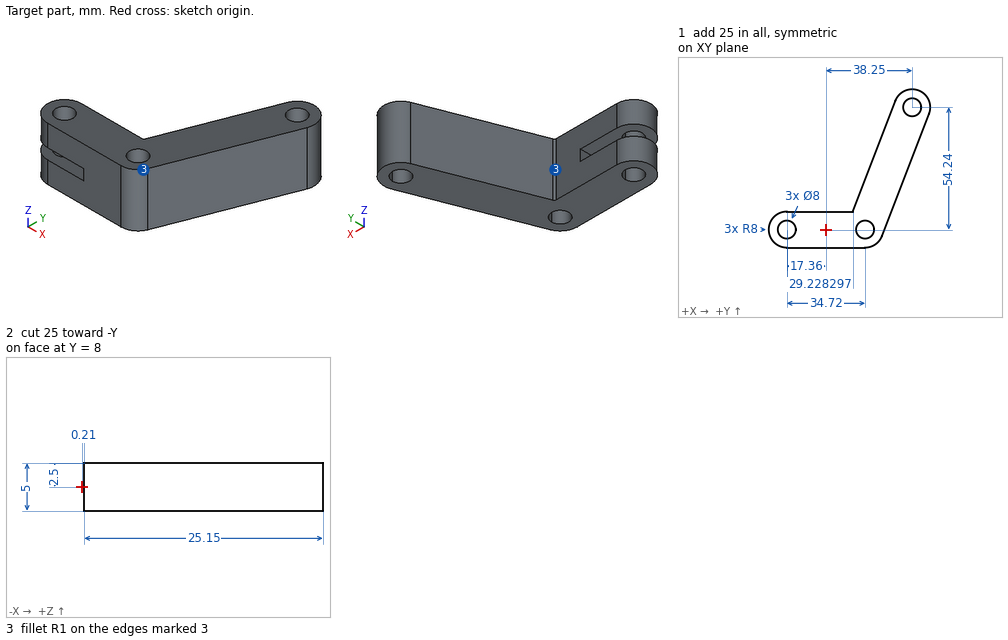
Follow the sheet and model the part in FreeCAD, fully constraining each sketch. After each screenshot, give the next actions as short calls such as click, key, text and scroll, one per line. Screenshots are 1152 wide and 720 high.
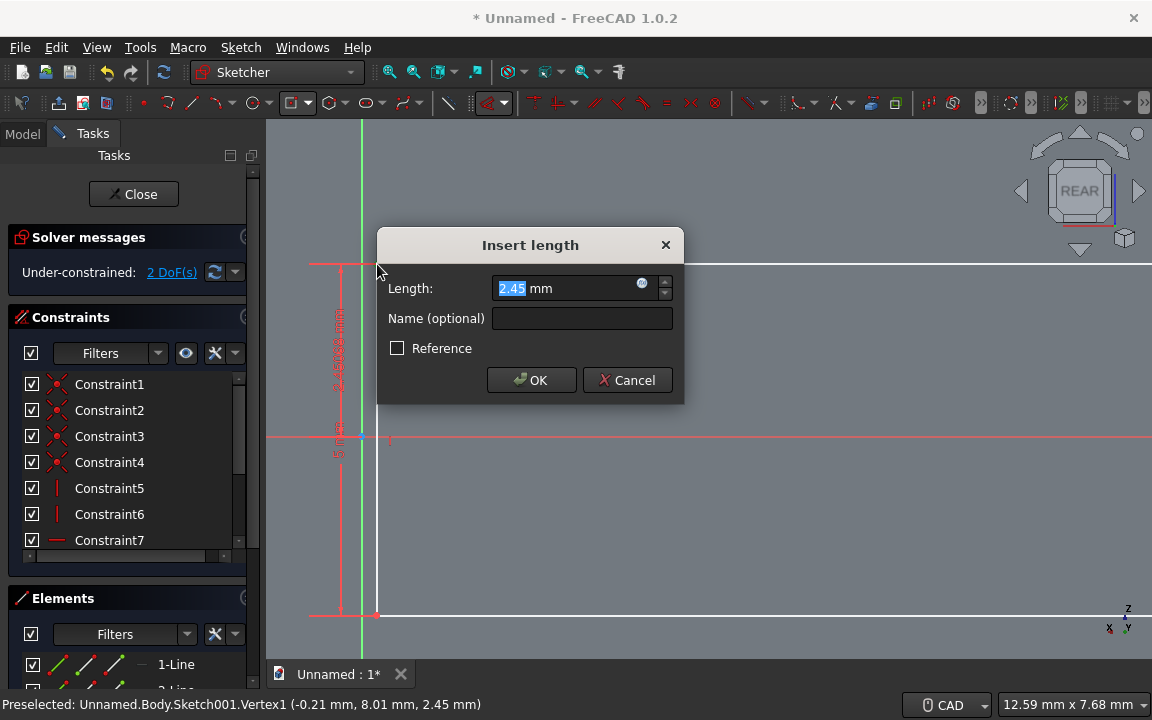
text(2.5)
key(Return)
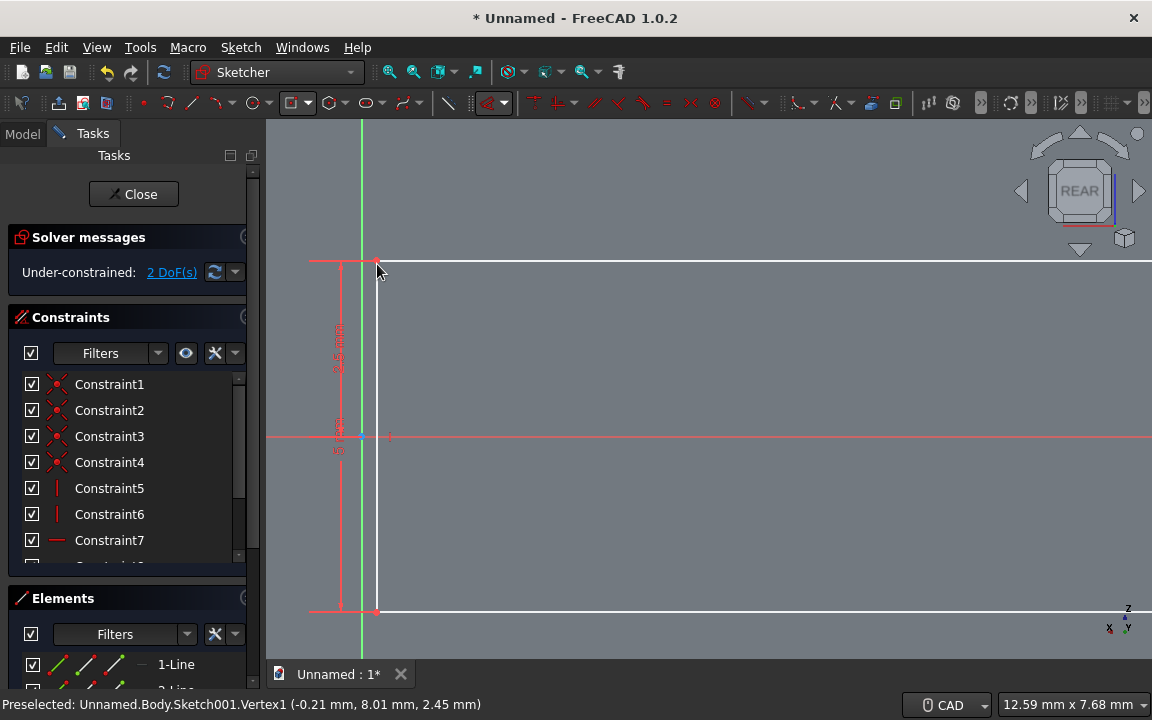
click(907, 612)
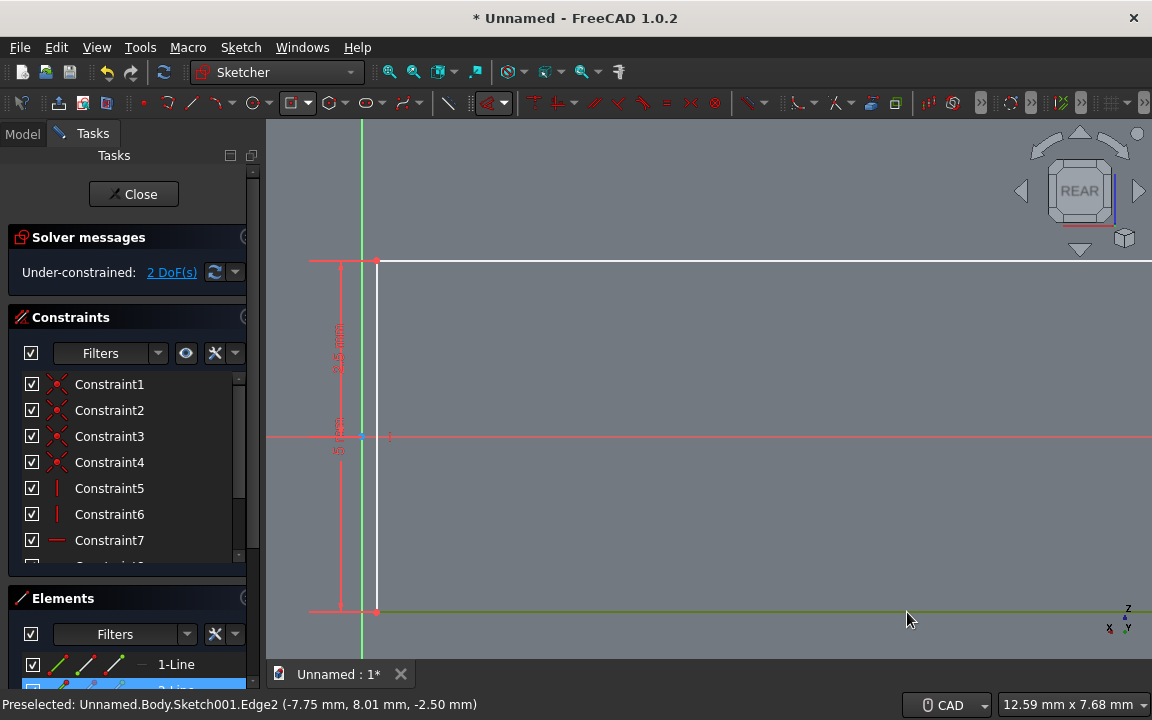
key(l)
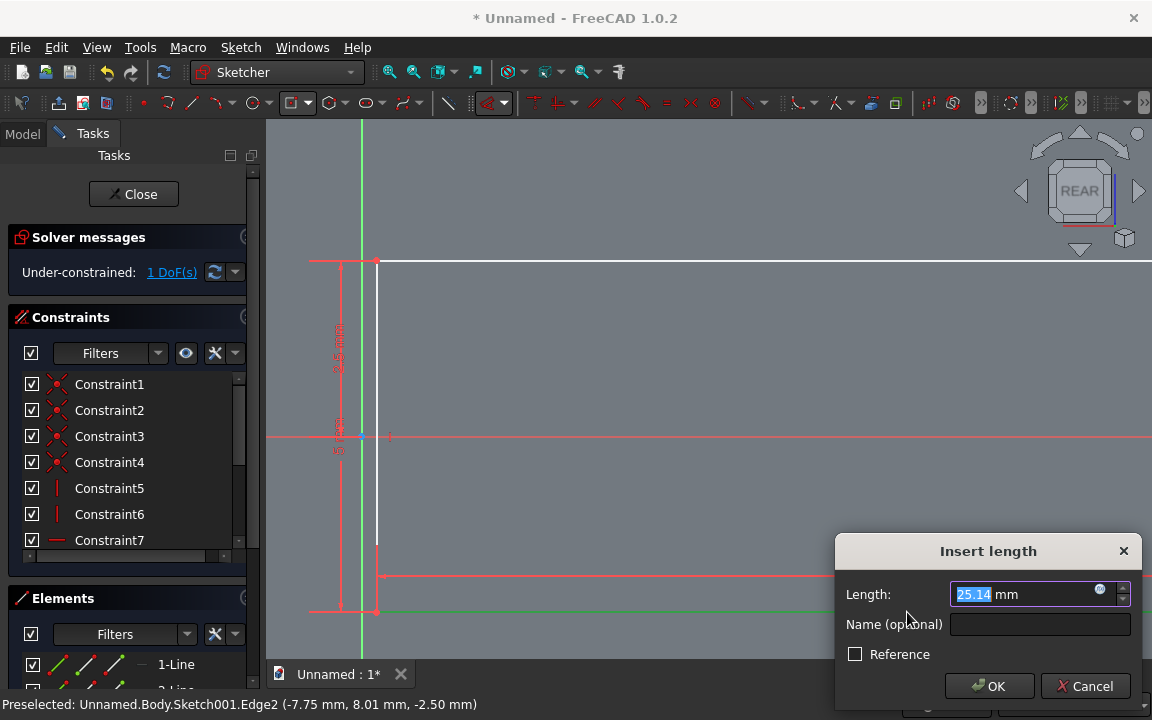
text(25.15)
key(Return)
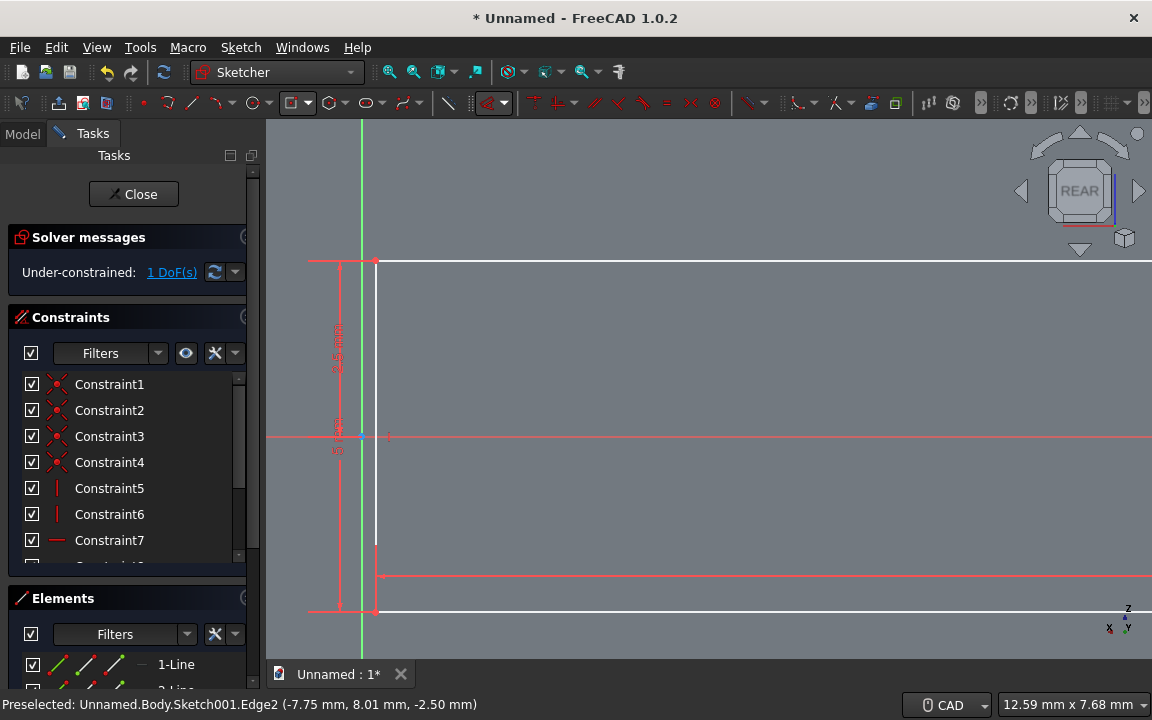
scroll(376, 261, up, 5)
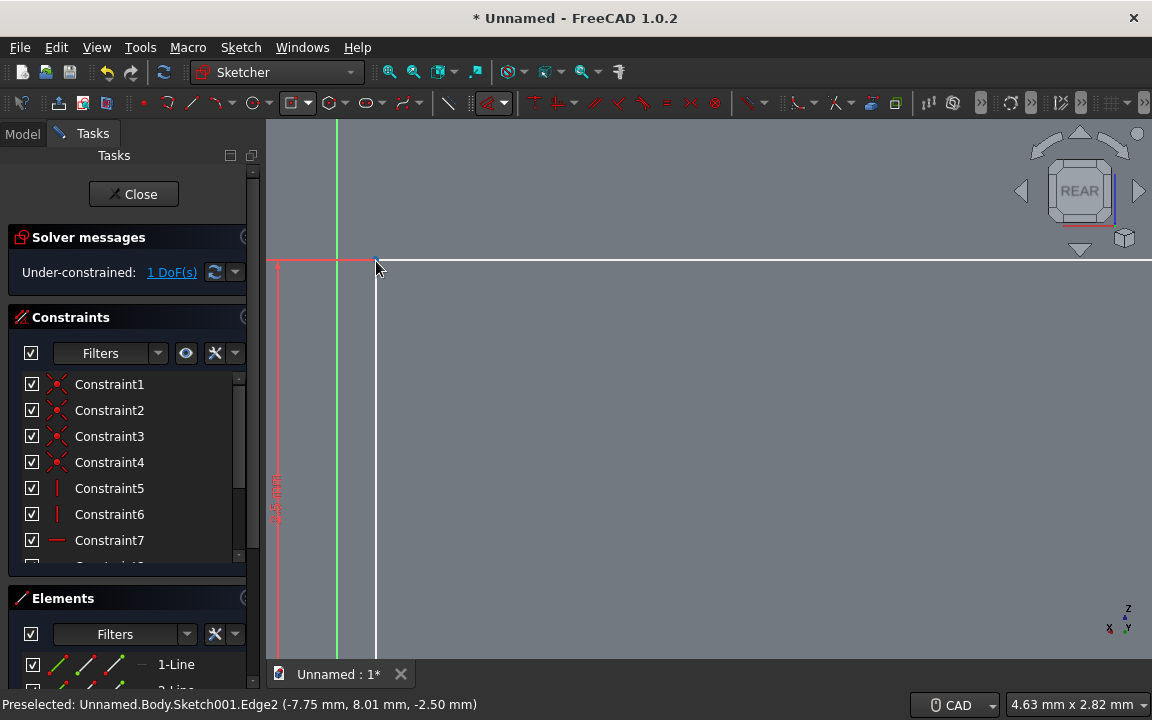
click(376, 260)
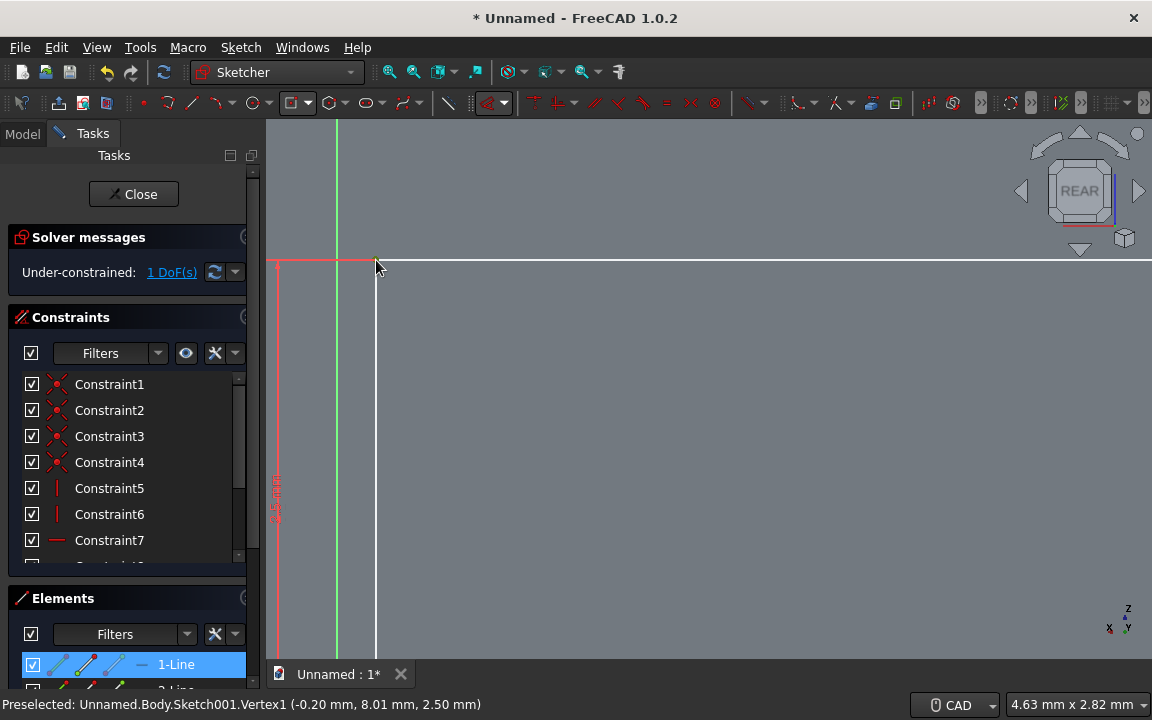
click(506, 104)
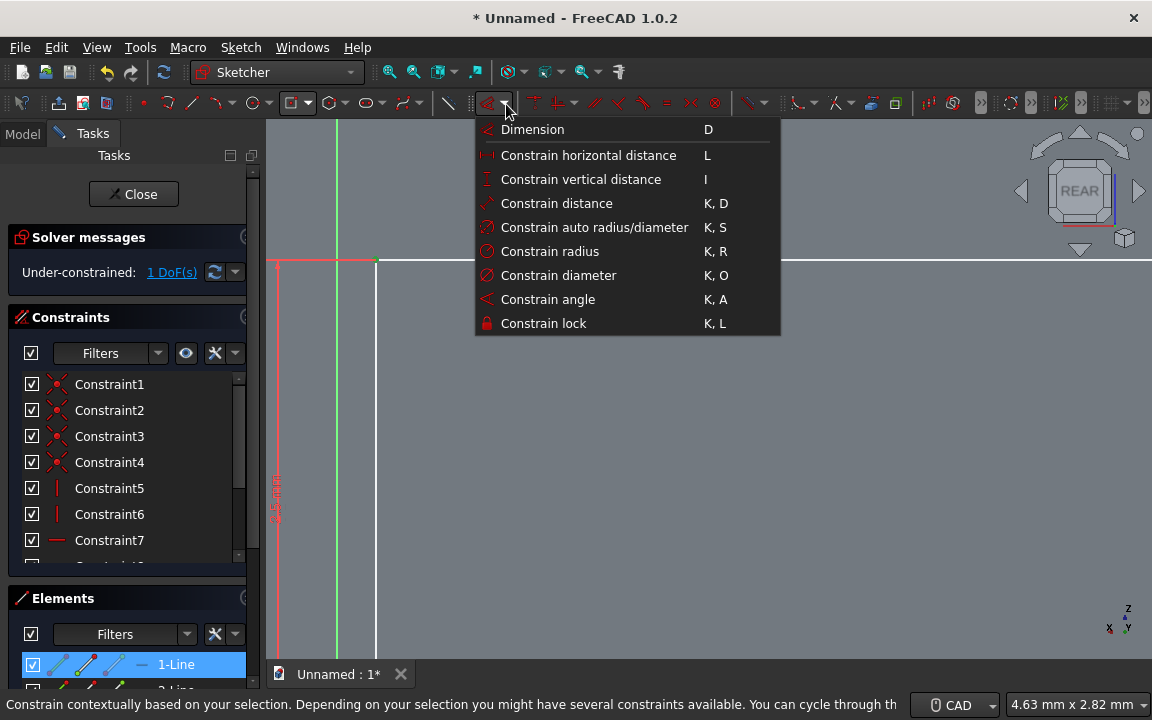
click(628, 155)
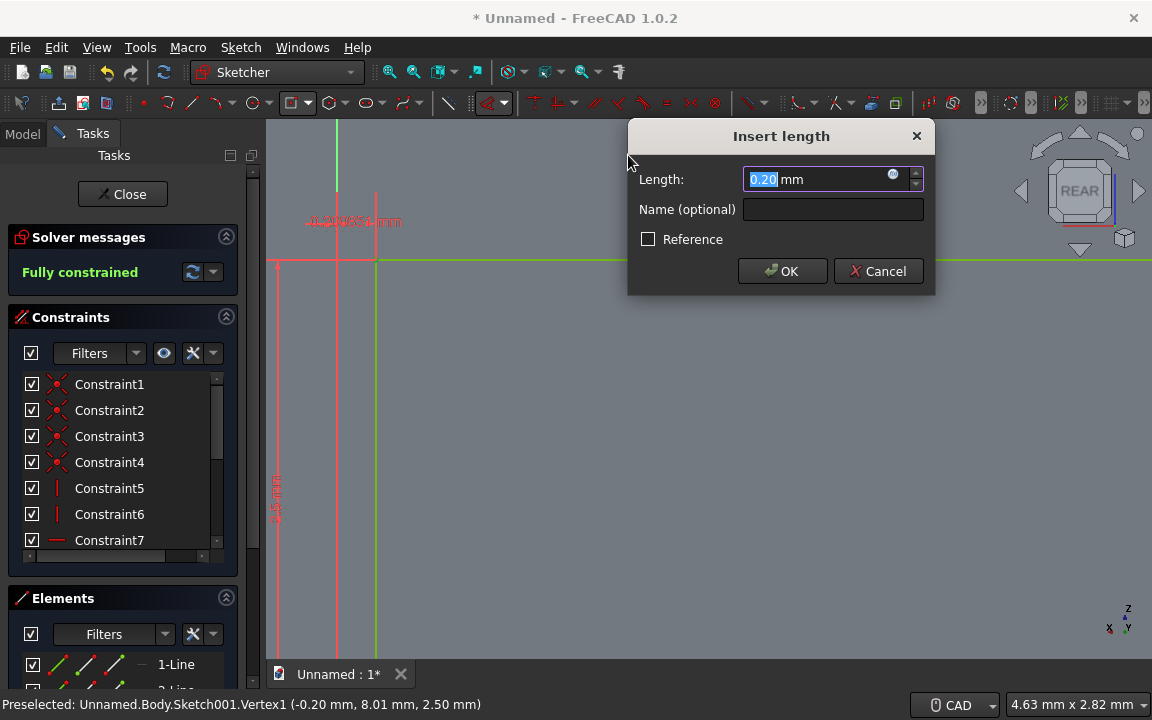
text(0.21)
key(Return)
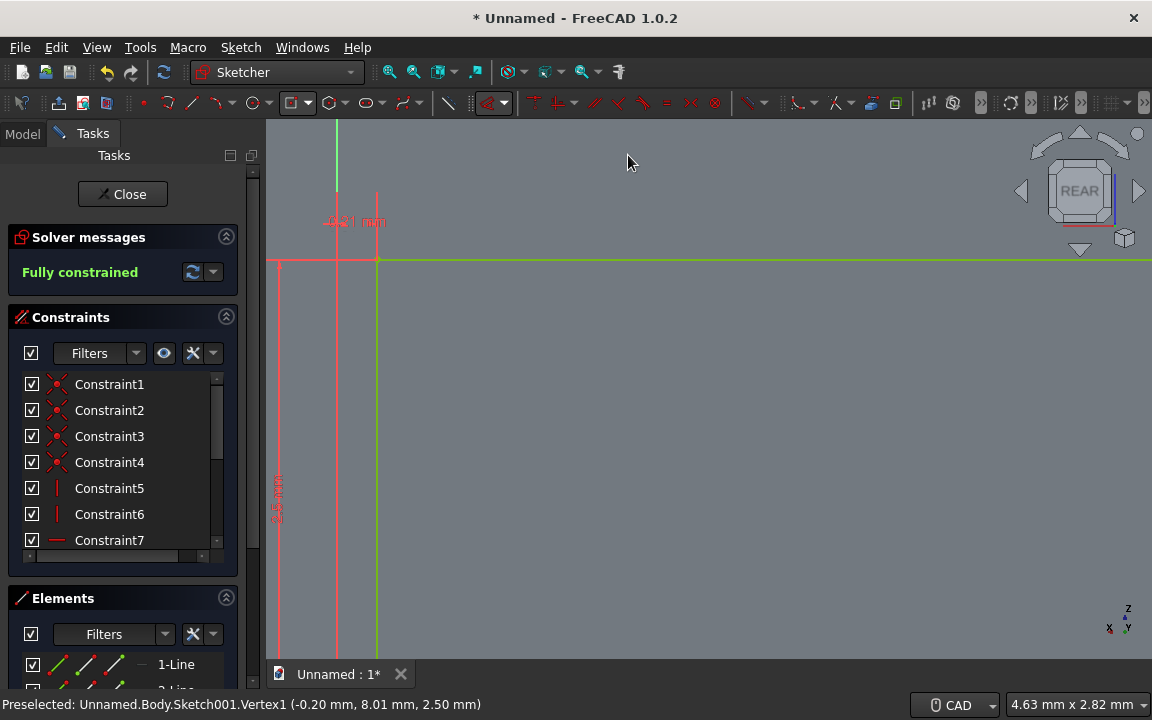
click(123, 194)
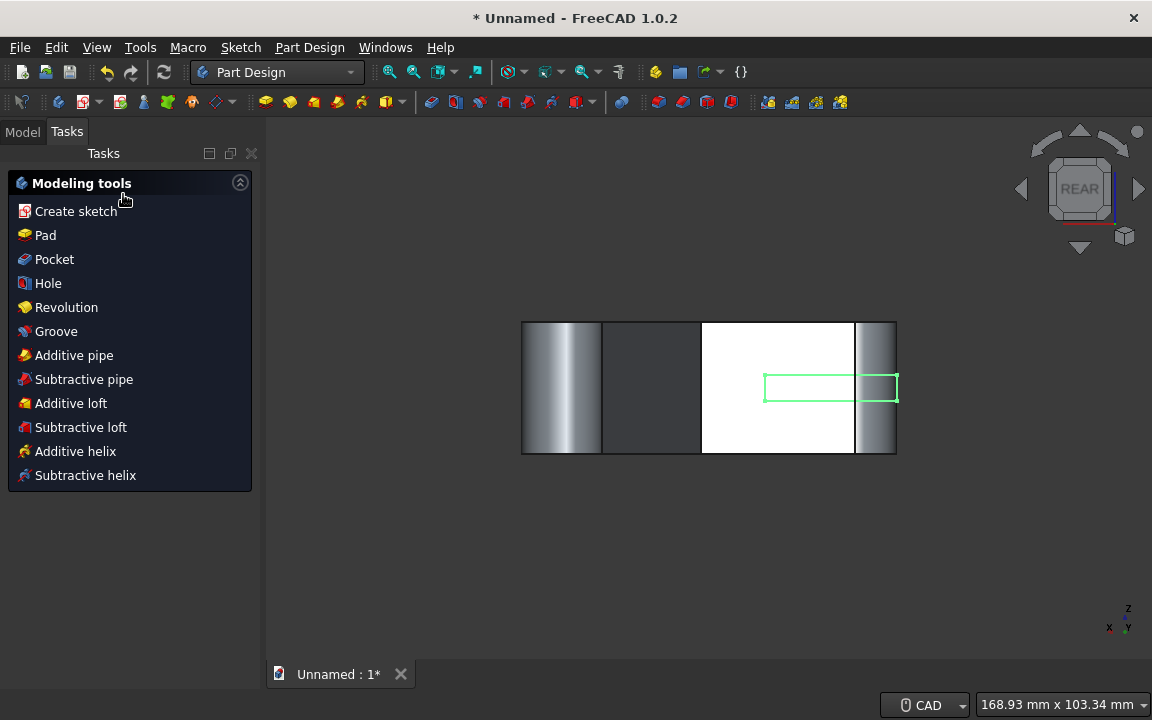
click(432, 102)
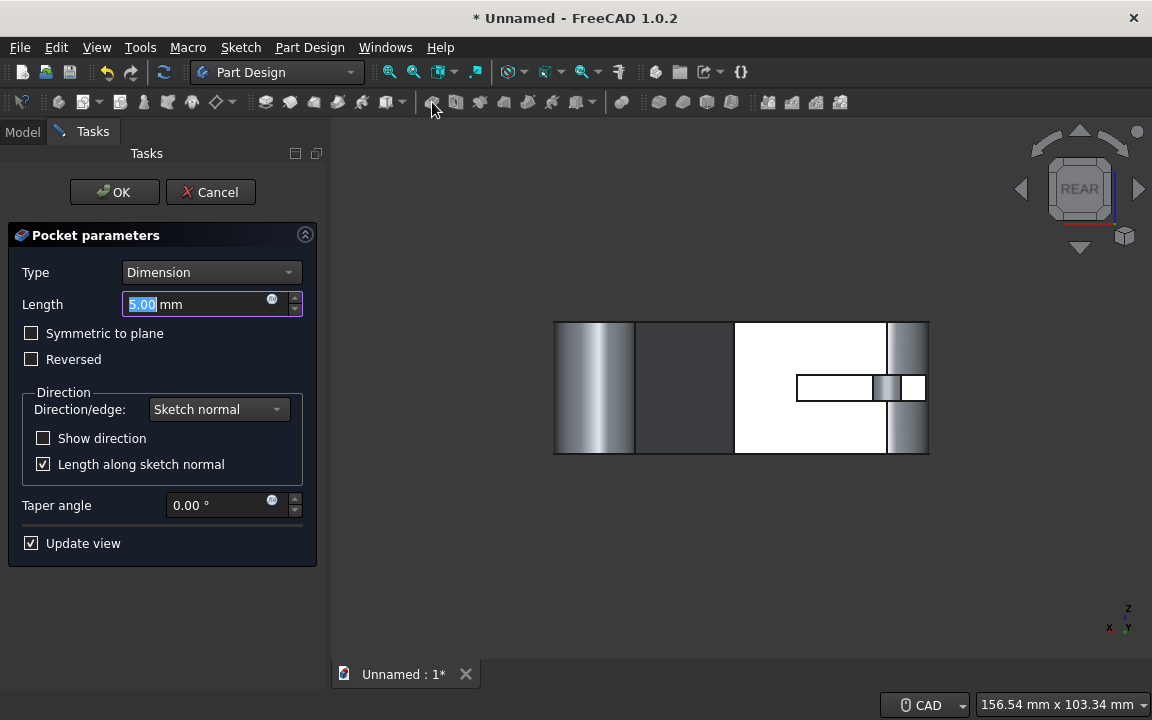
text(25)
key(Tab)